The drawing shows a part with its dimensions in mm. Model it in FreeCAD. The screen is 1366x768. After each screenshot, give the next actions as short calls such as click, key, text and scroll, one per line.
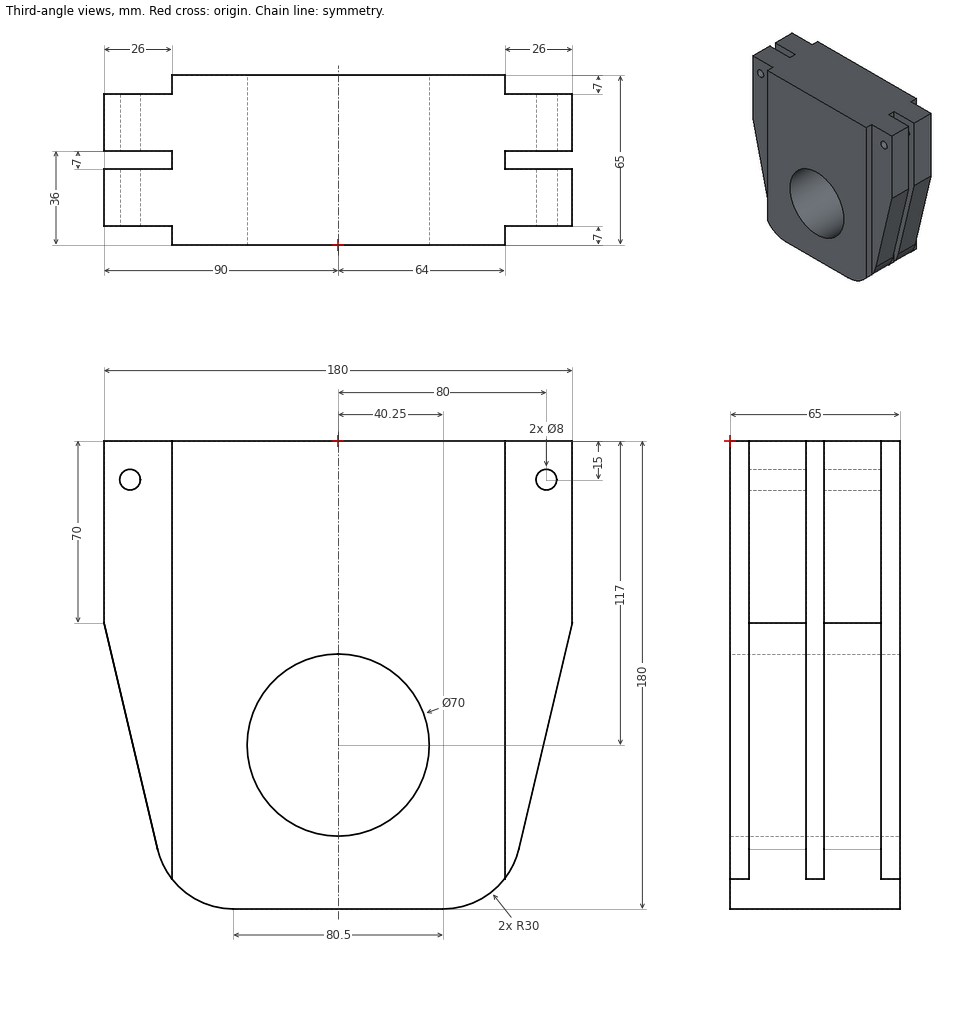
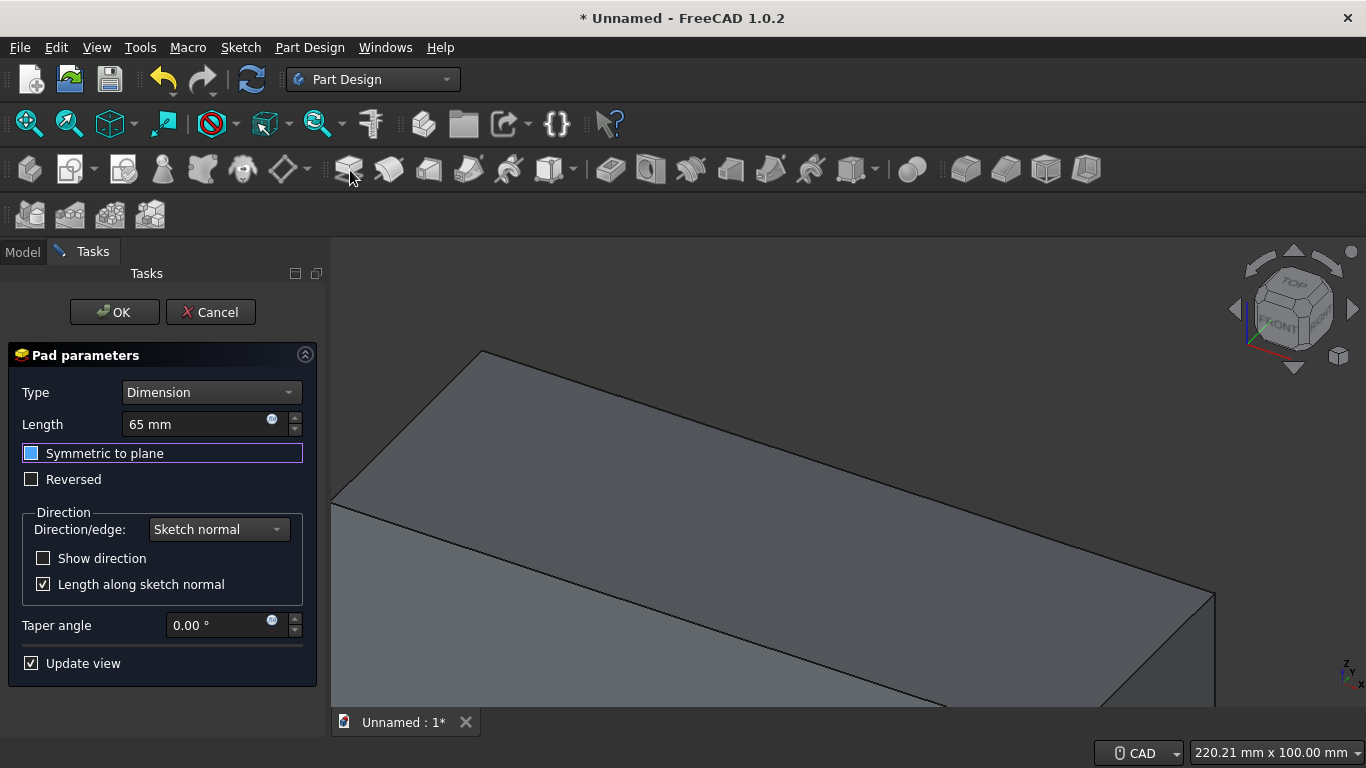
click(30, 479)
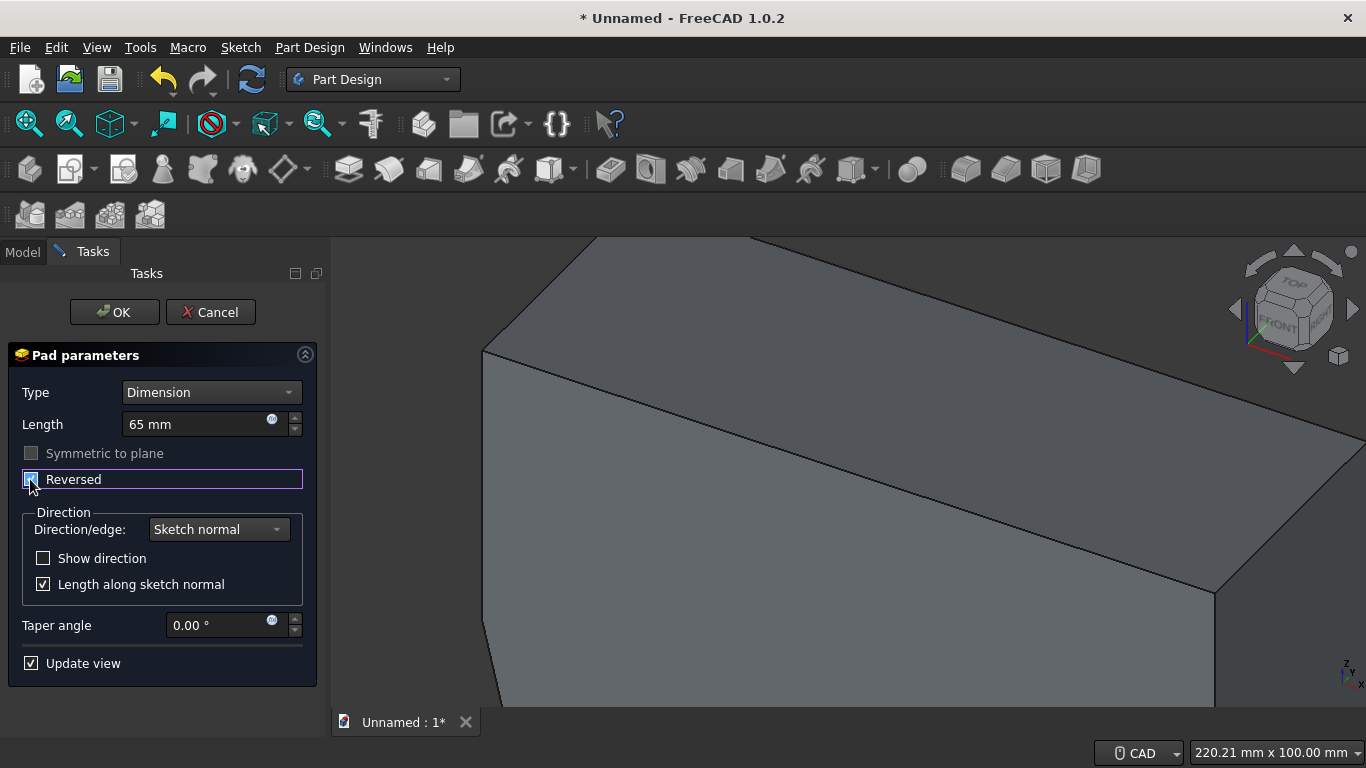
click(115, 312)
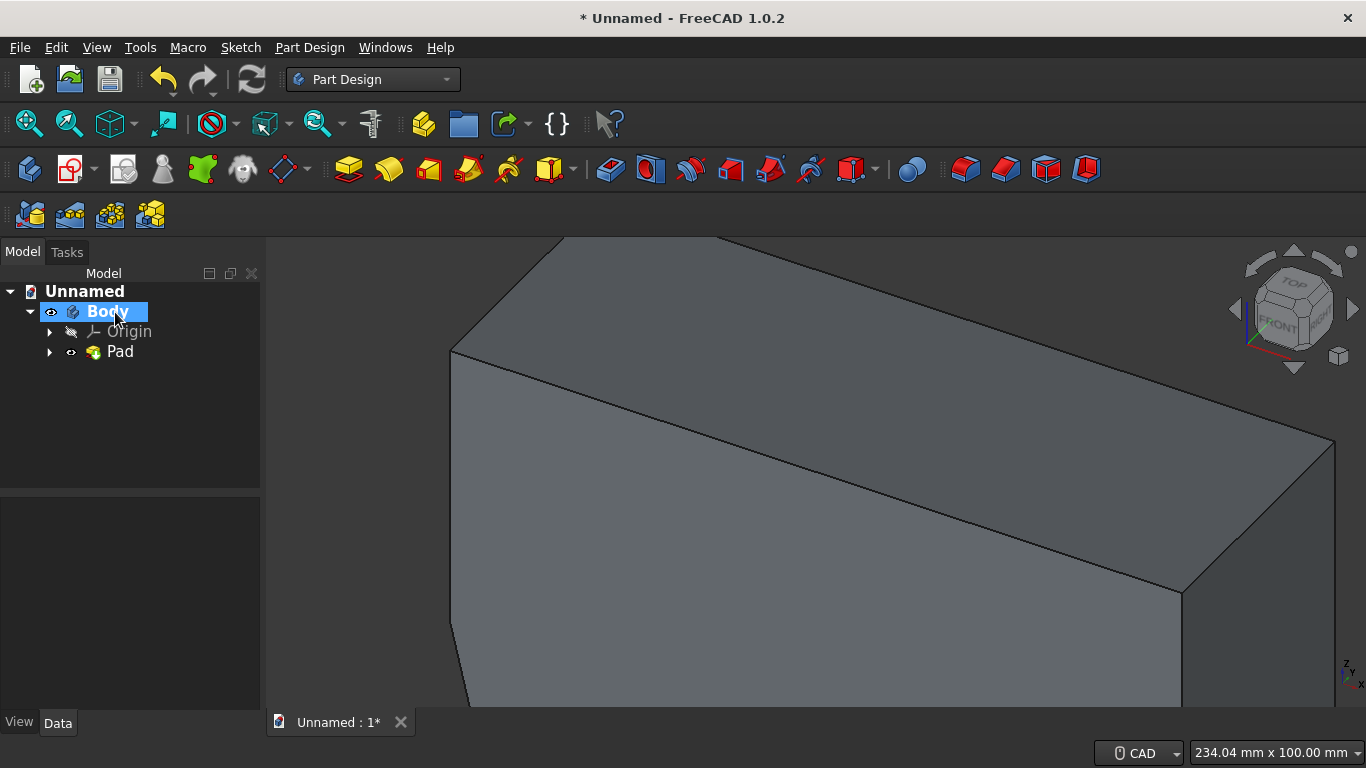
click(30, 124)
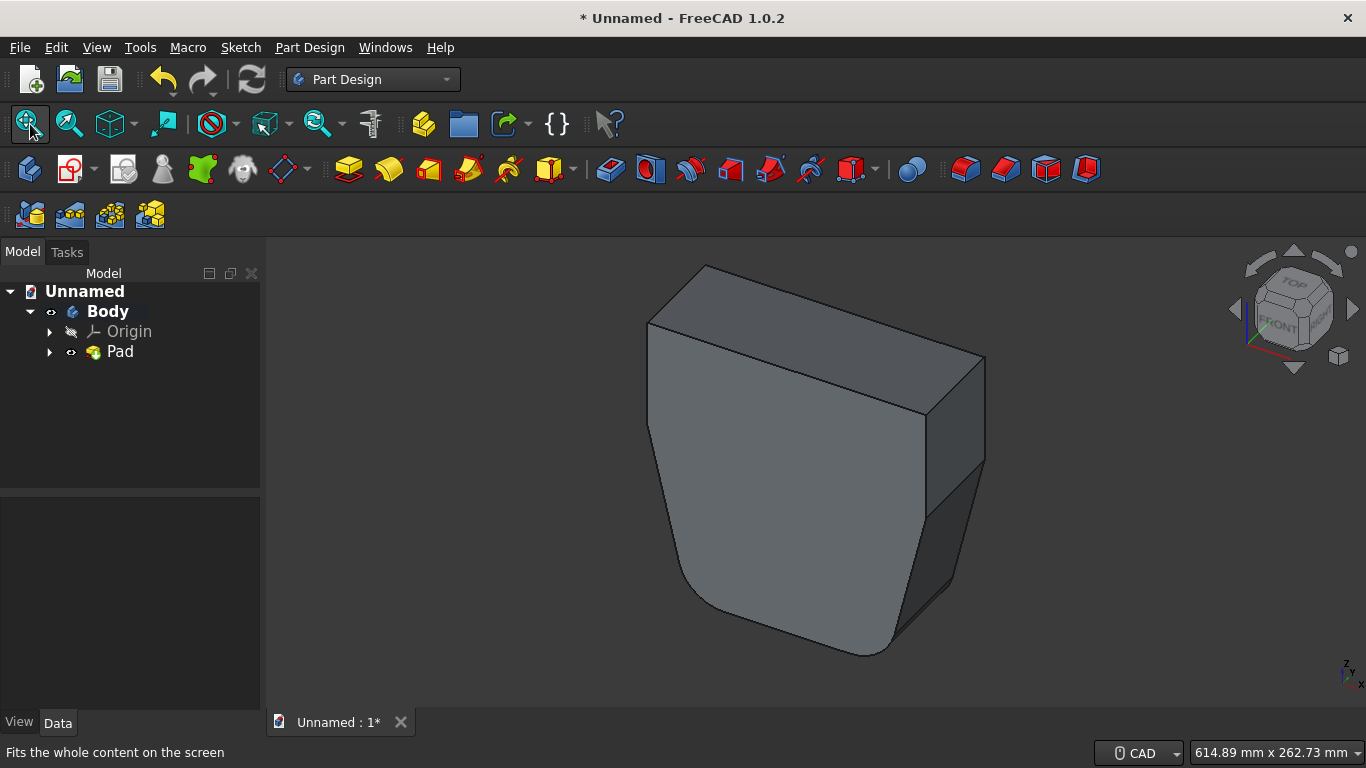
key(4)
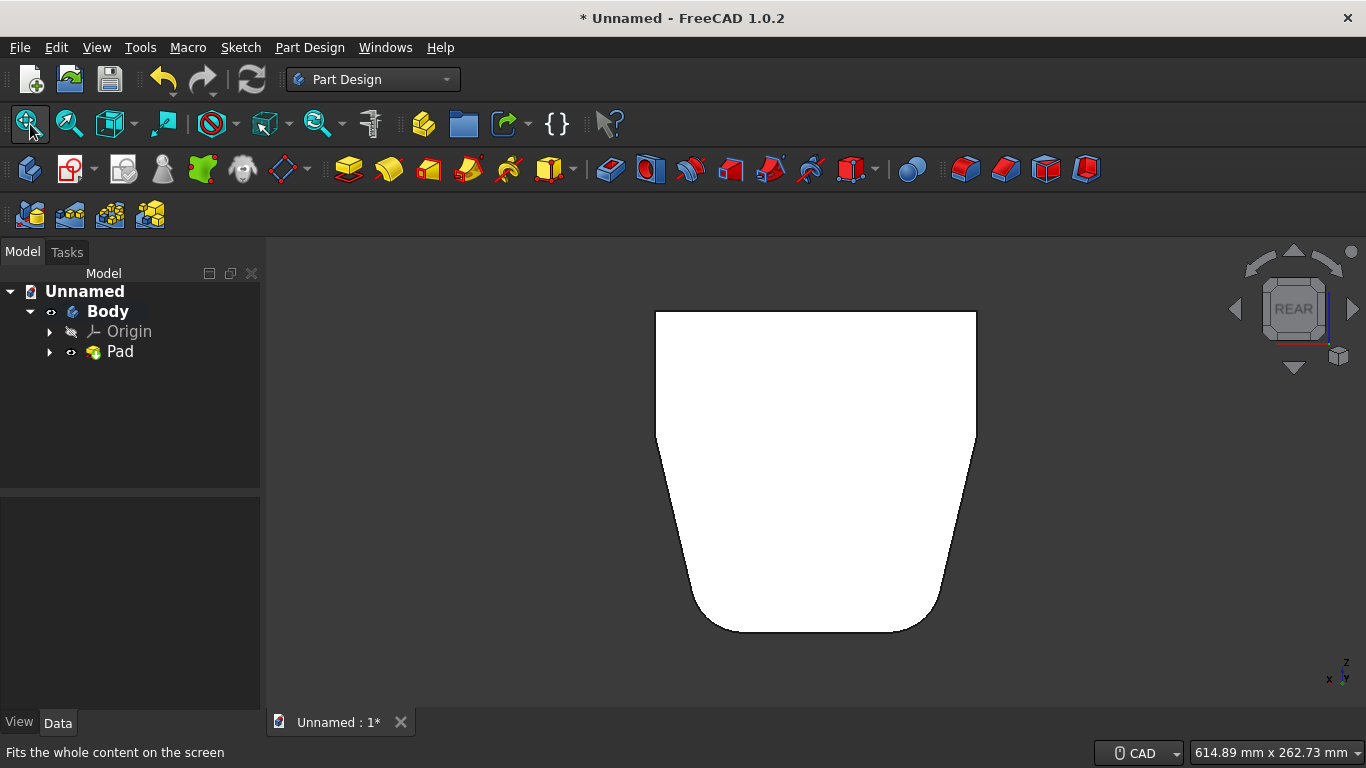
click(816, 471)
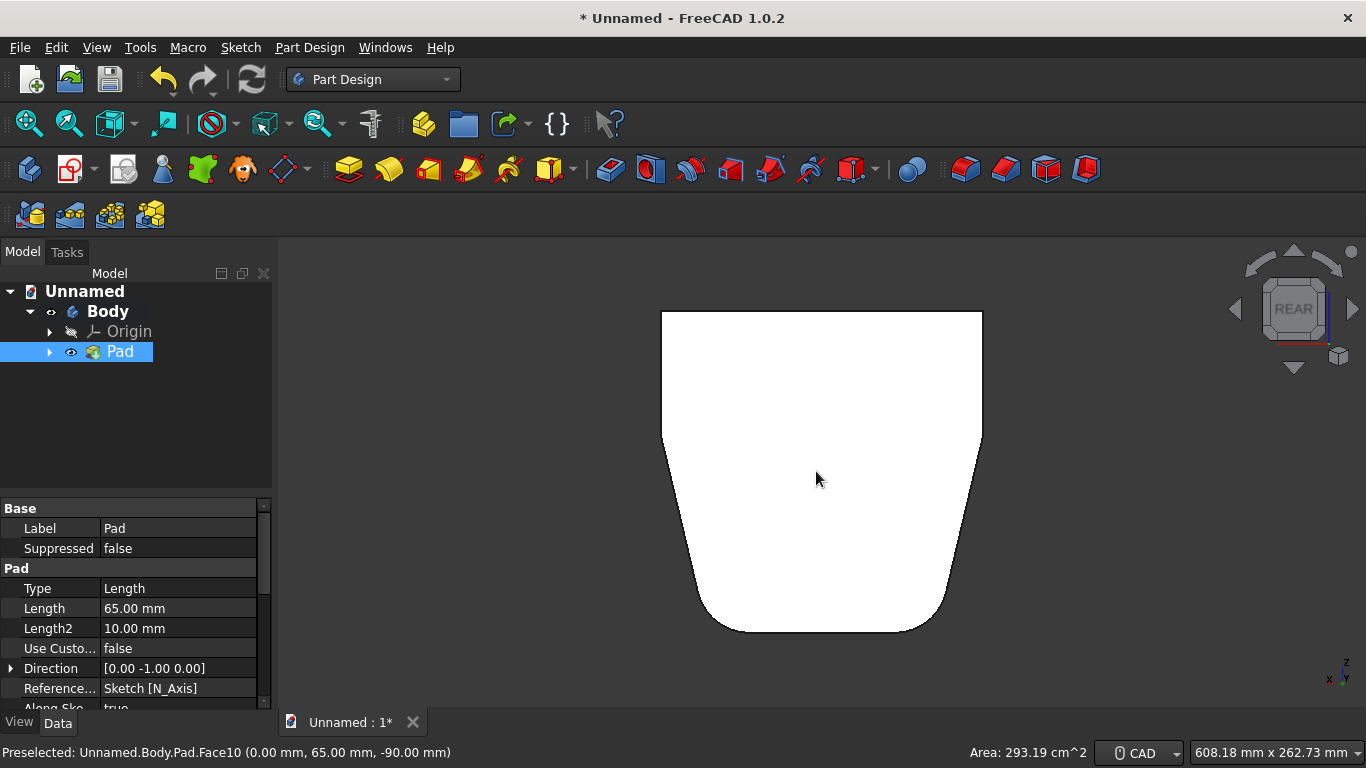
click(70, 170)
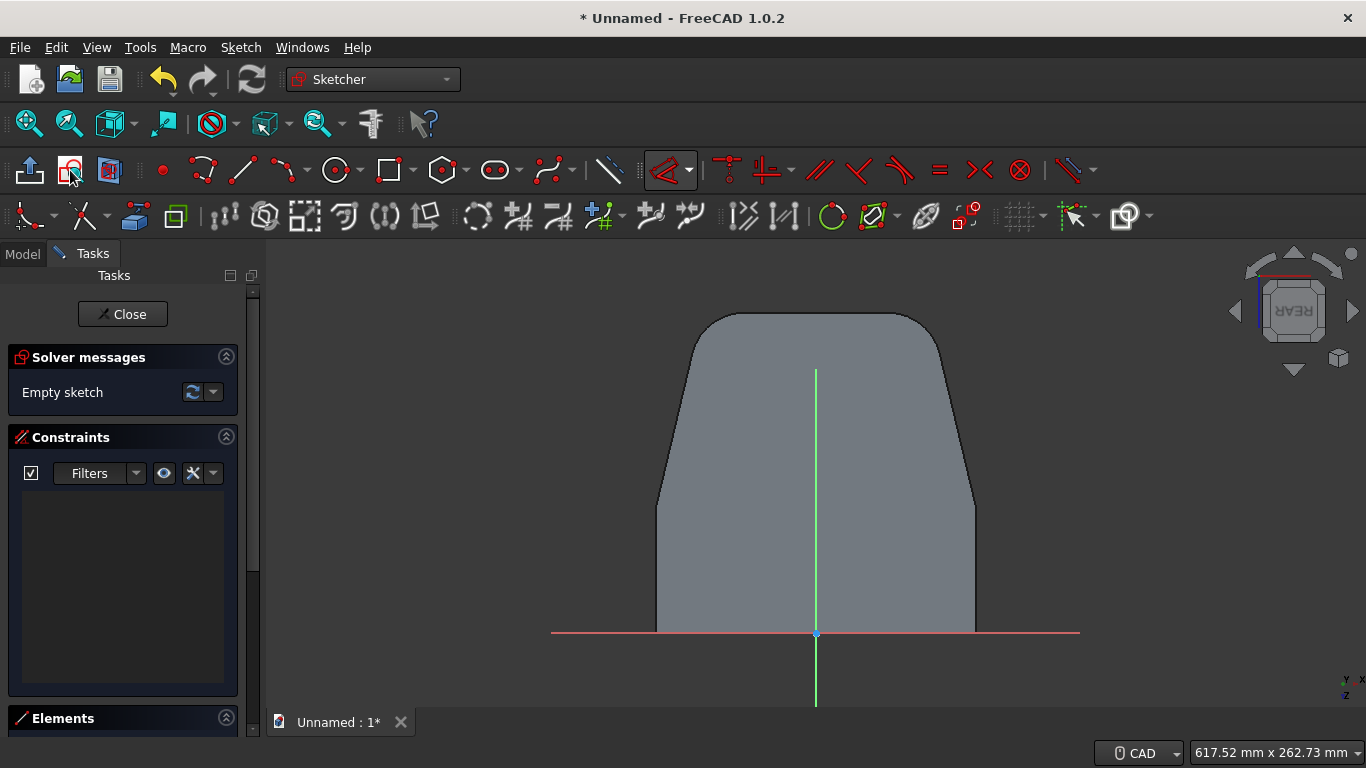
click(336, 170)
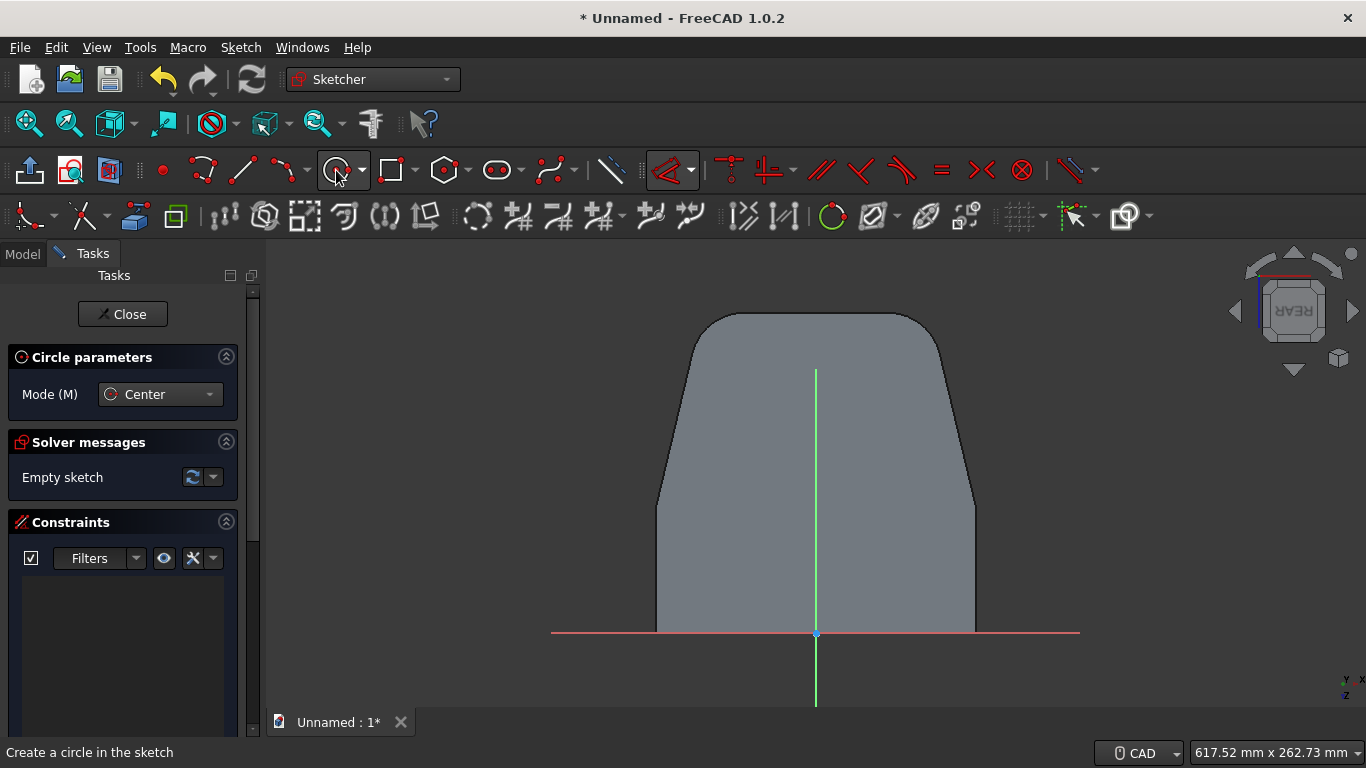
click(816, 425)
move(860, 381)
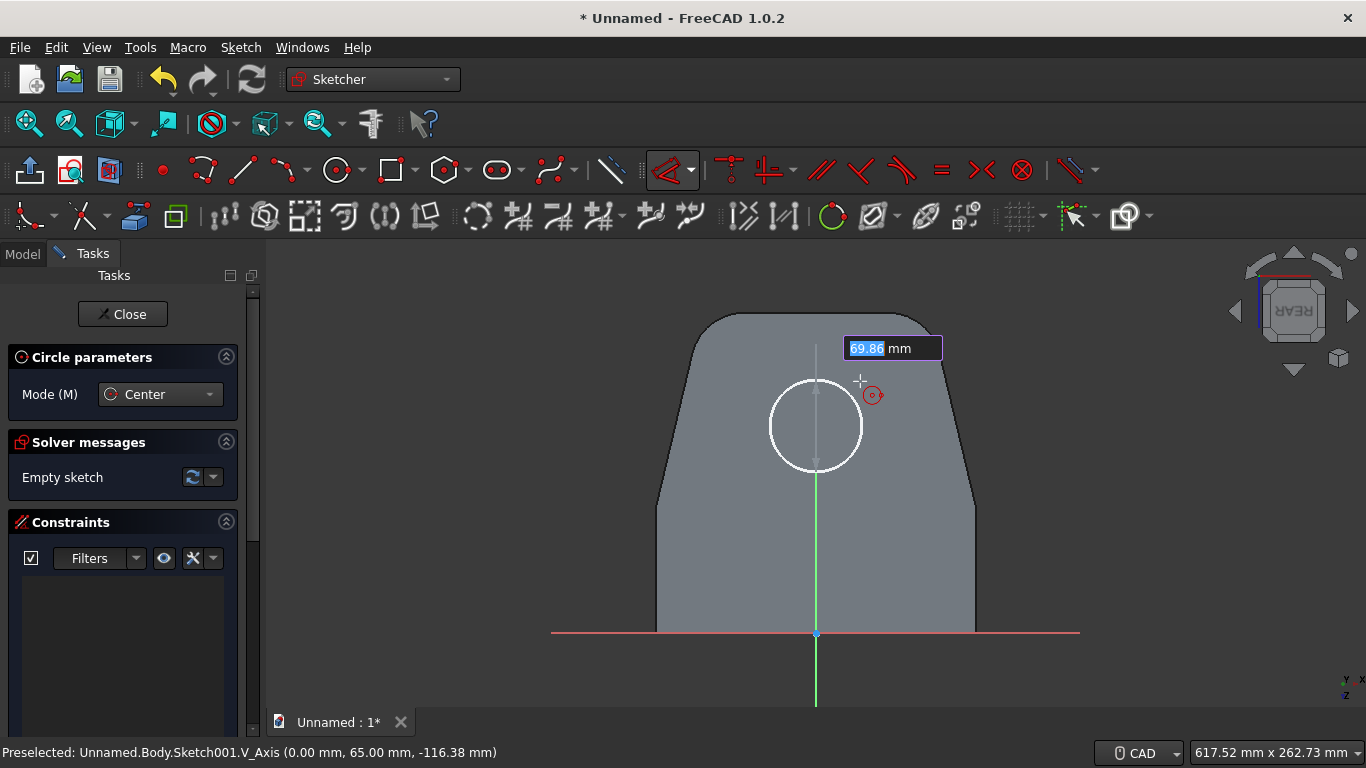
text(70)
key(Return)
key(Escape)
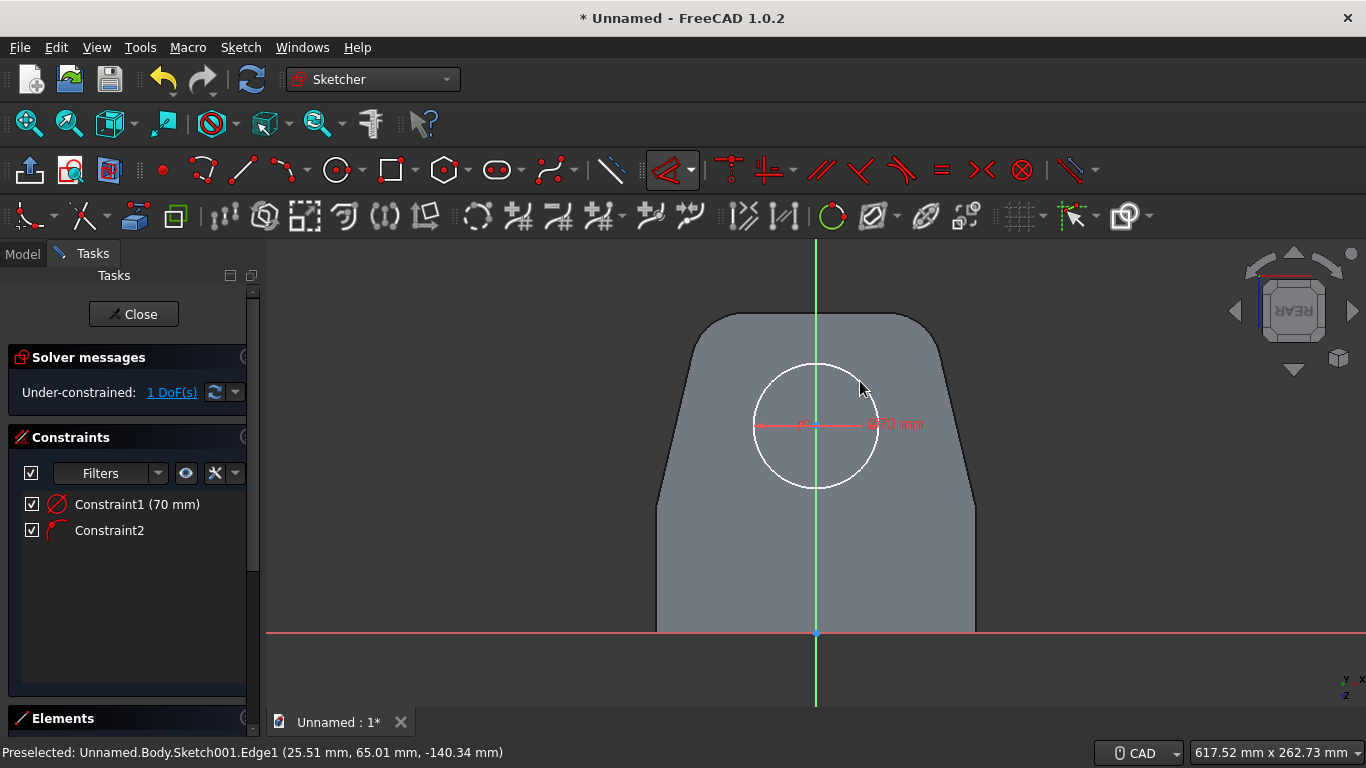
click(816, 426)